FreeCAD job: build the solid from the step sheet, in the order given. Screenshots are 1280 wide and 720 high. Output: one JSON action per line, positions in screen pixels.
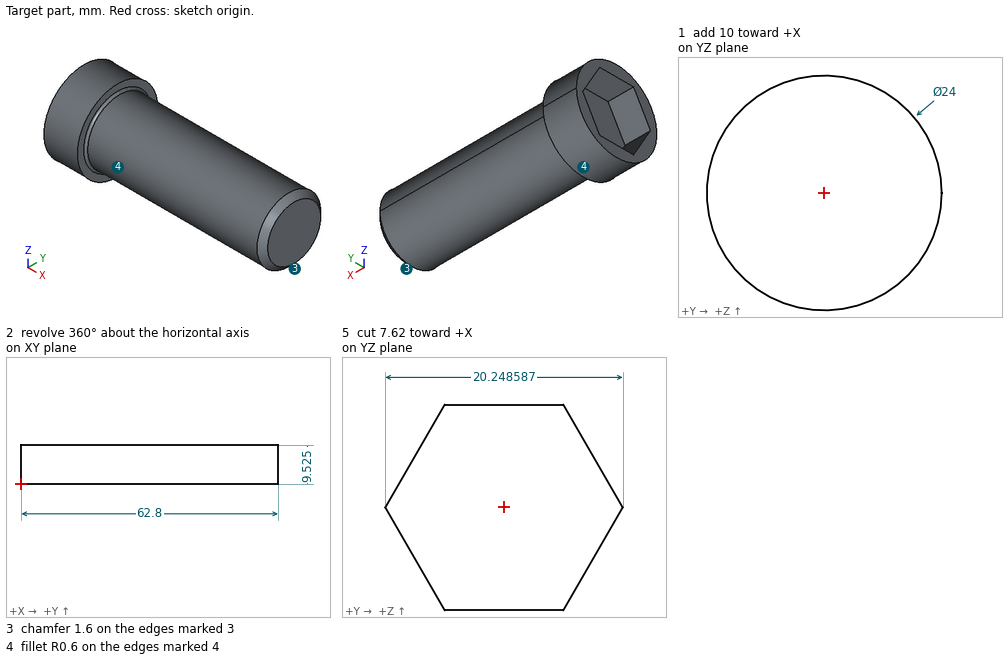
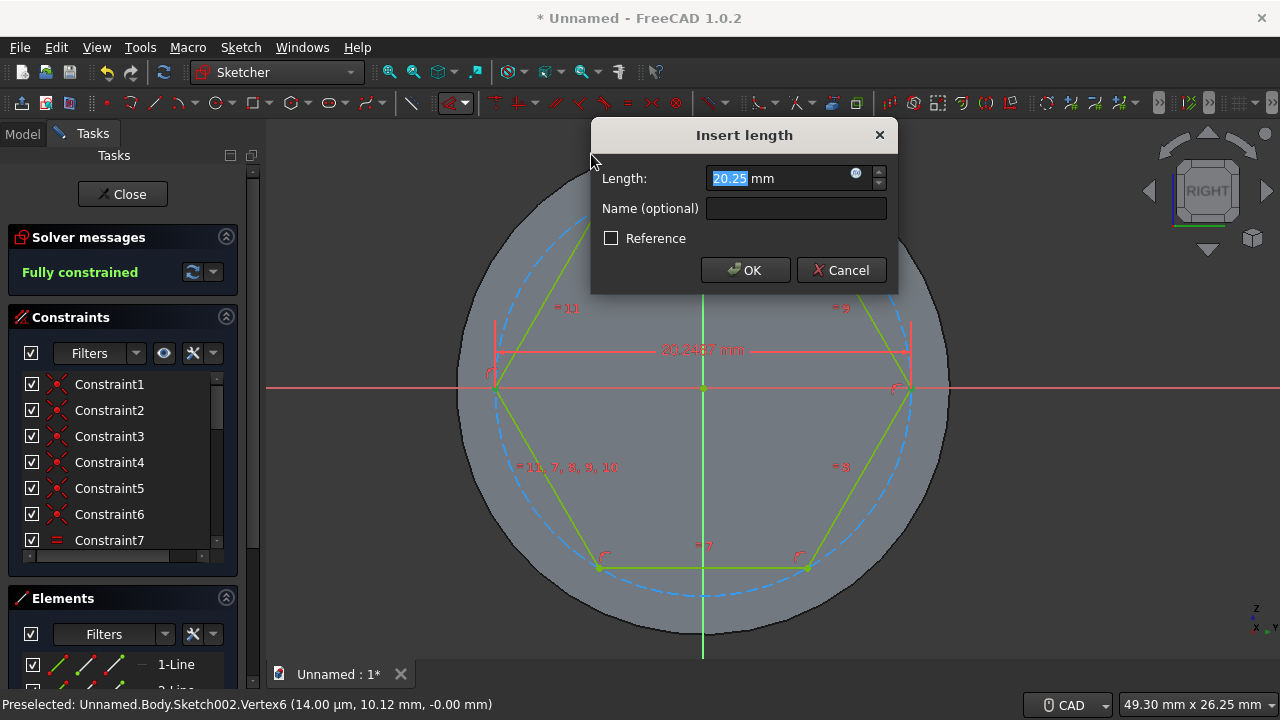
{"action": "type", "text": "20.248587"}
{"action": "key", "text": "Return"}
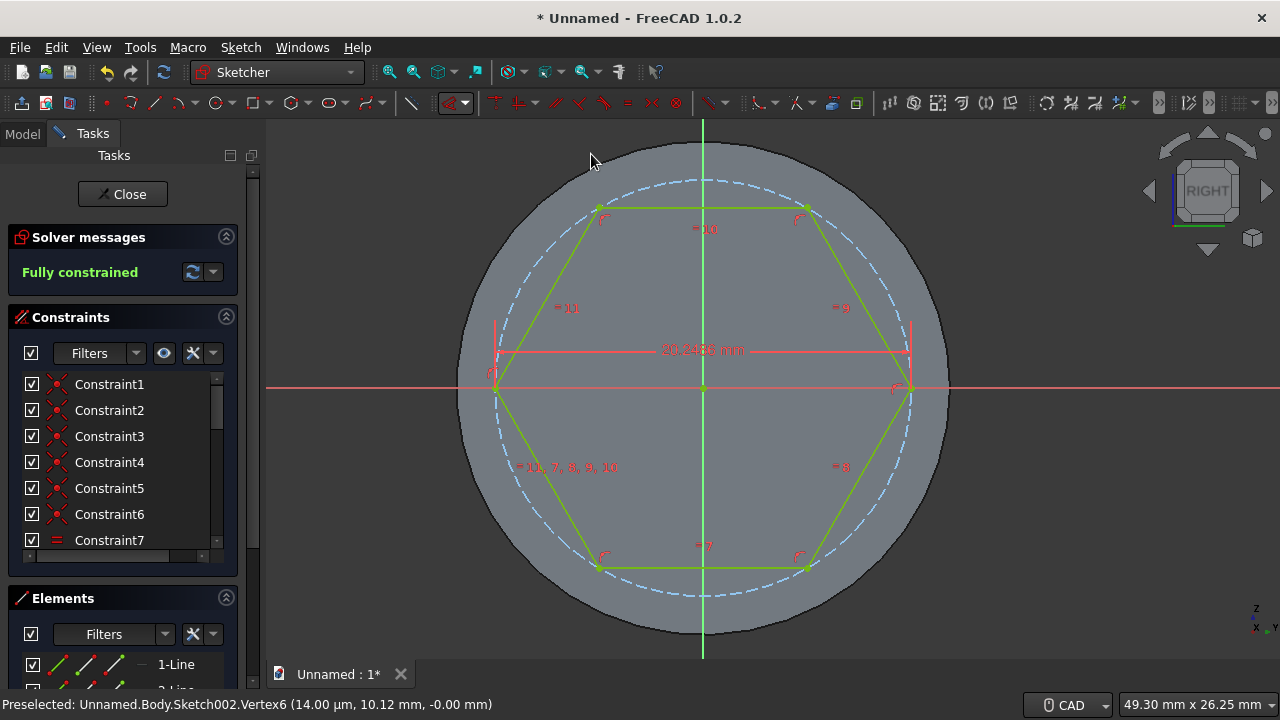
{"action": "left_click", "coordinate": [123, 194]}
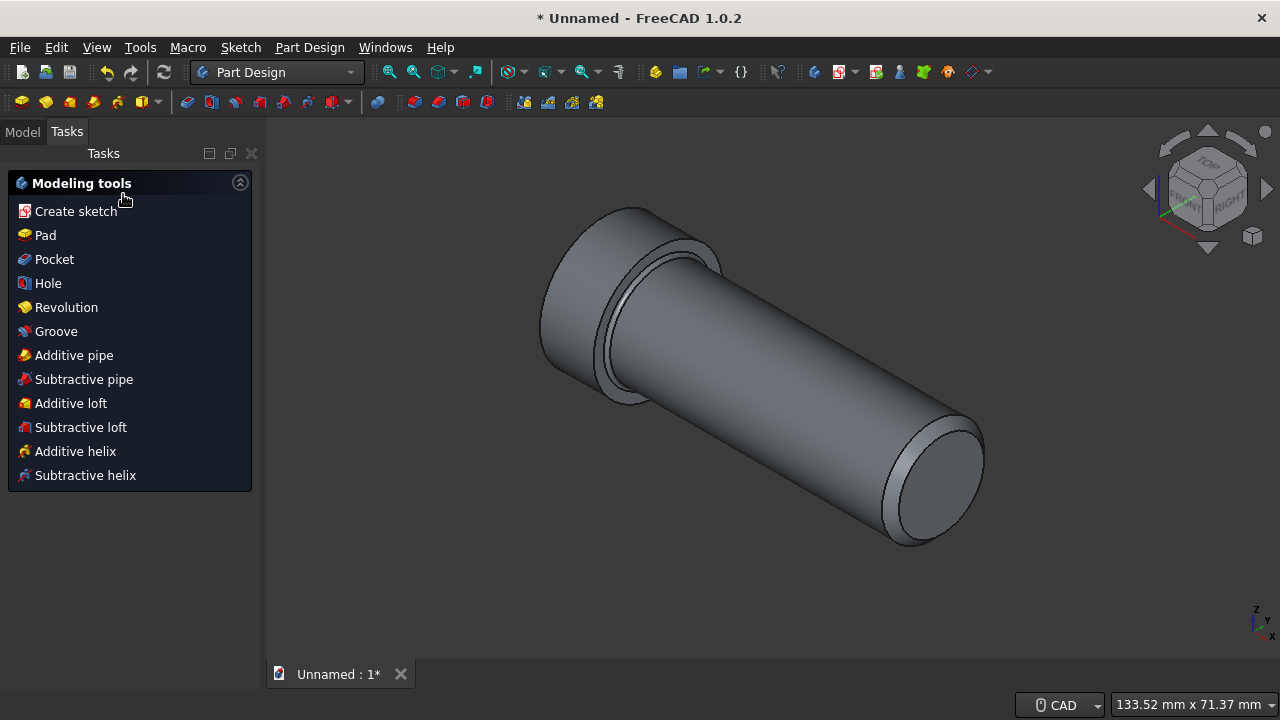
{"action": "left_click", "coordinate": [188, 102]}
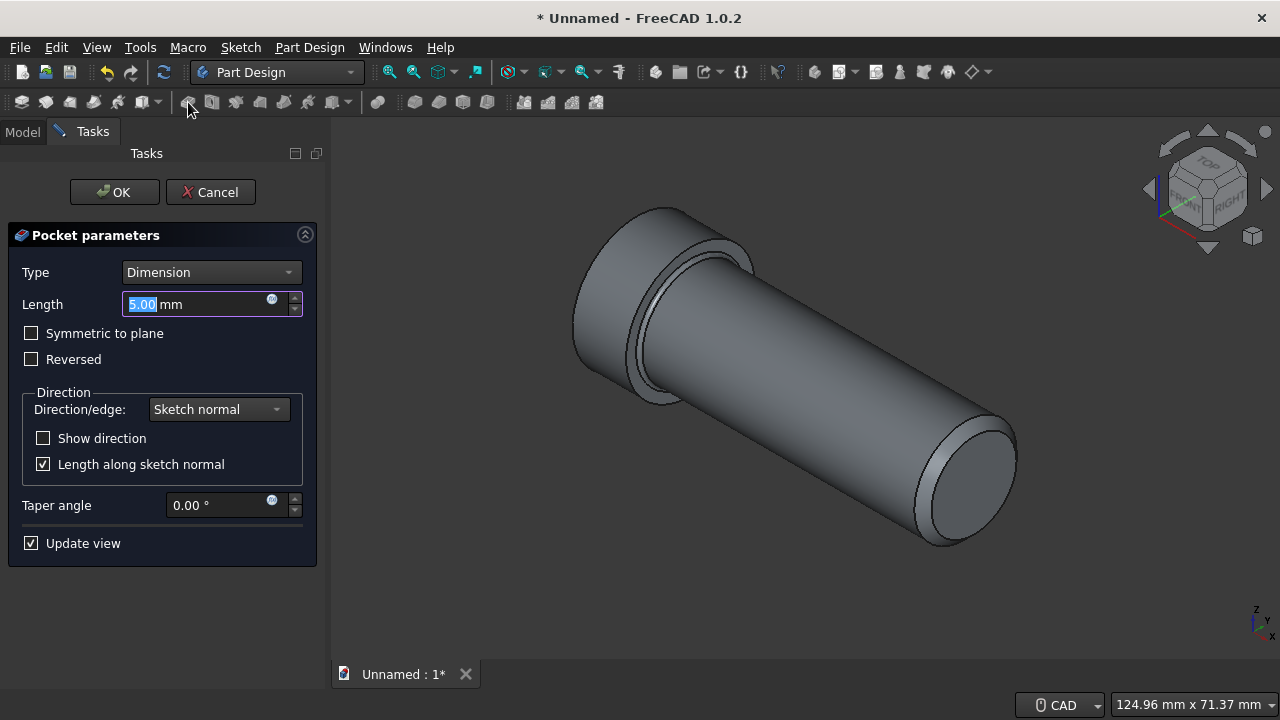
{"action": "type", "text": "7.62"}
{"action": "key", "text": "Tab"}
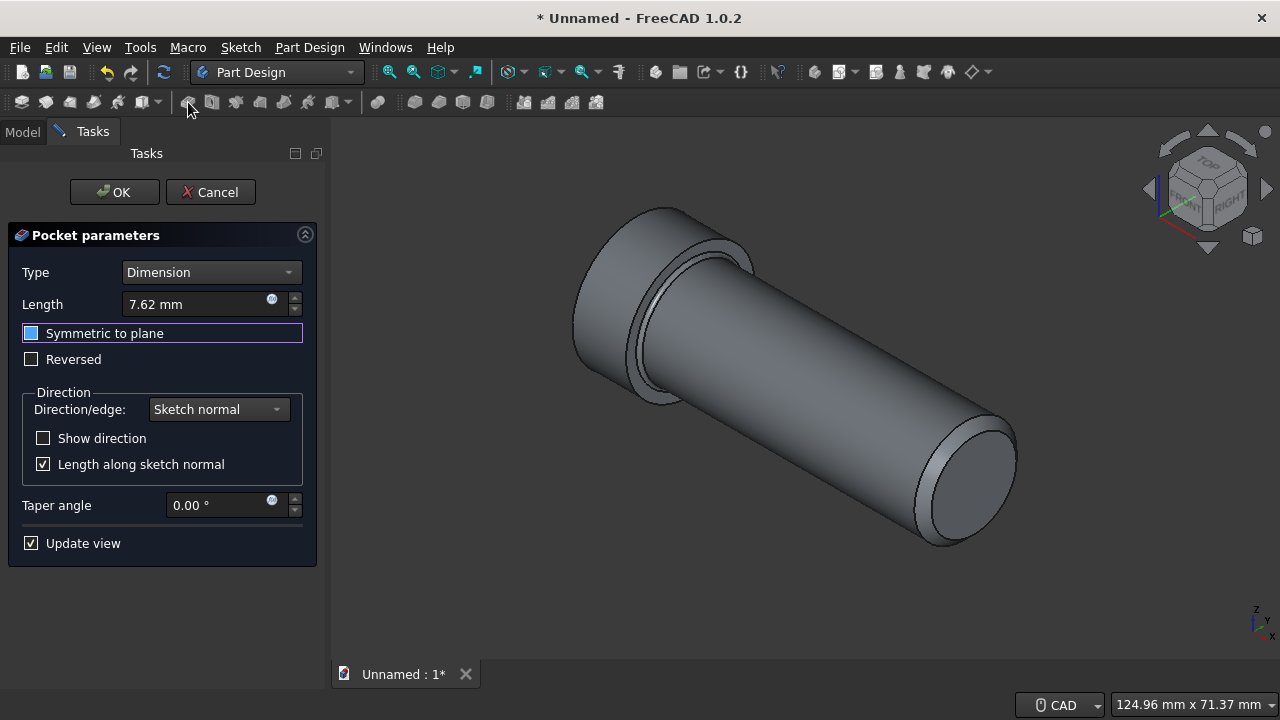
{"action": "left_click", "coordinate": [30, 359]}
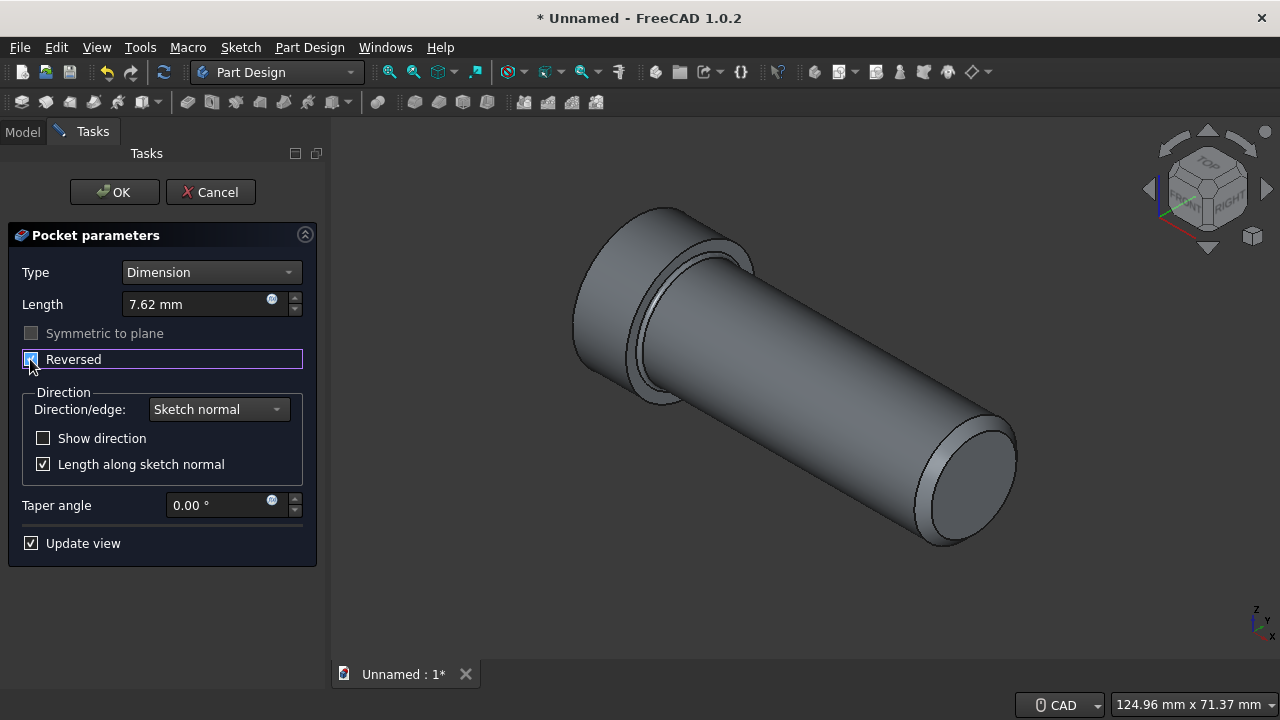
{"action": "left_click", "coordinate": [115, 192]}